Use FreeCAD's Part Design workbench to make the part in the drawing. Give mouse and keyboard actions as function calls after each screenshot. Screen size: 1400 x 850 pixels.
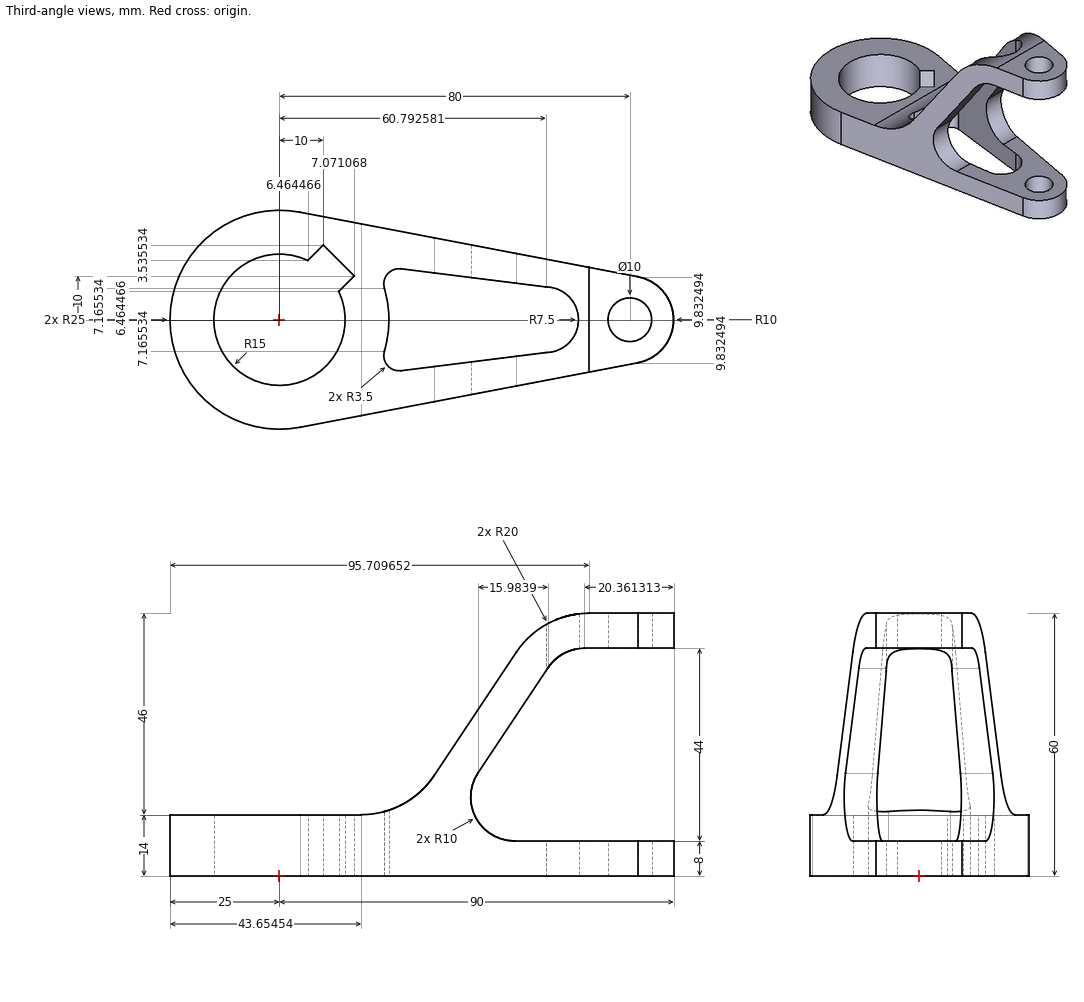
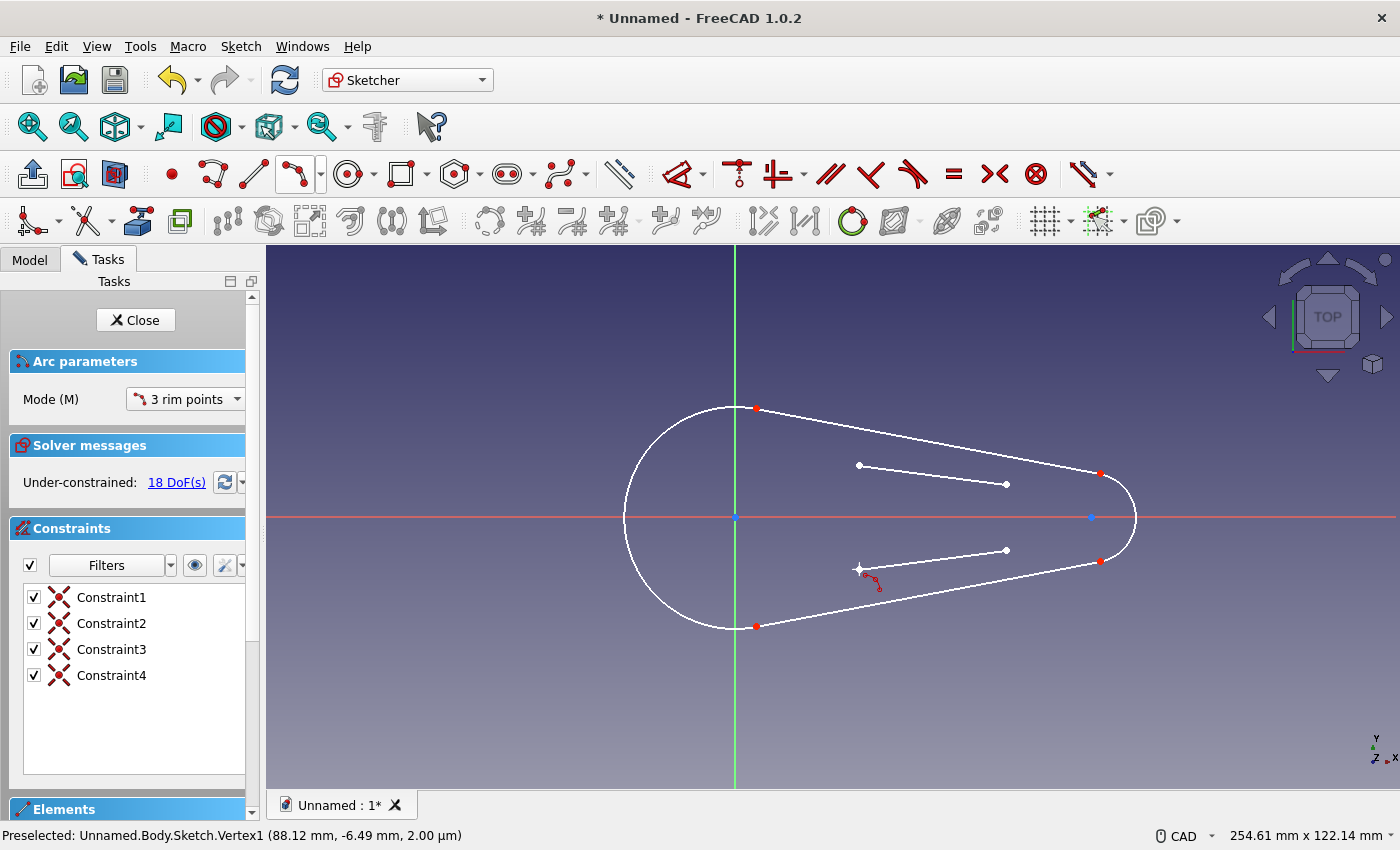
click(1006, 485)
click(1006, 551)
click(1033, 537)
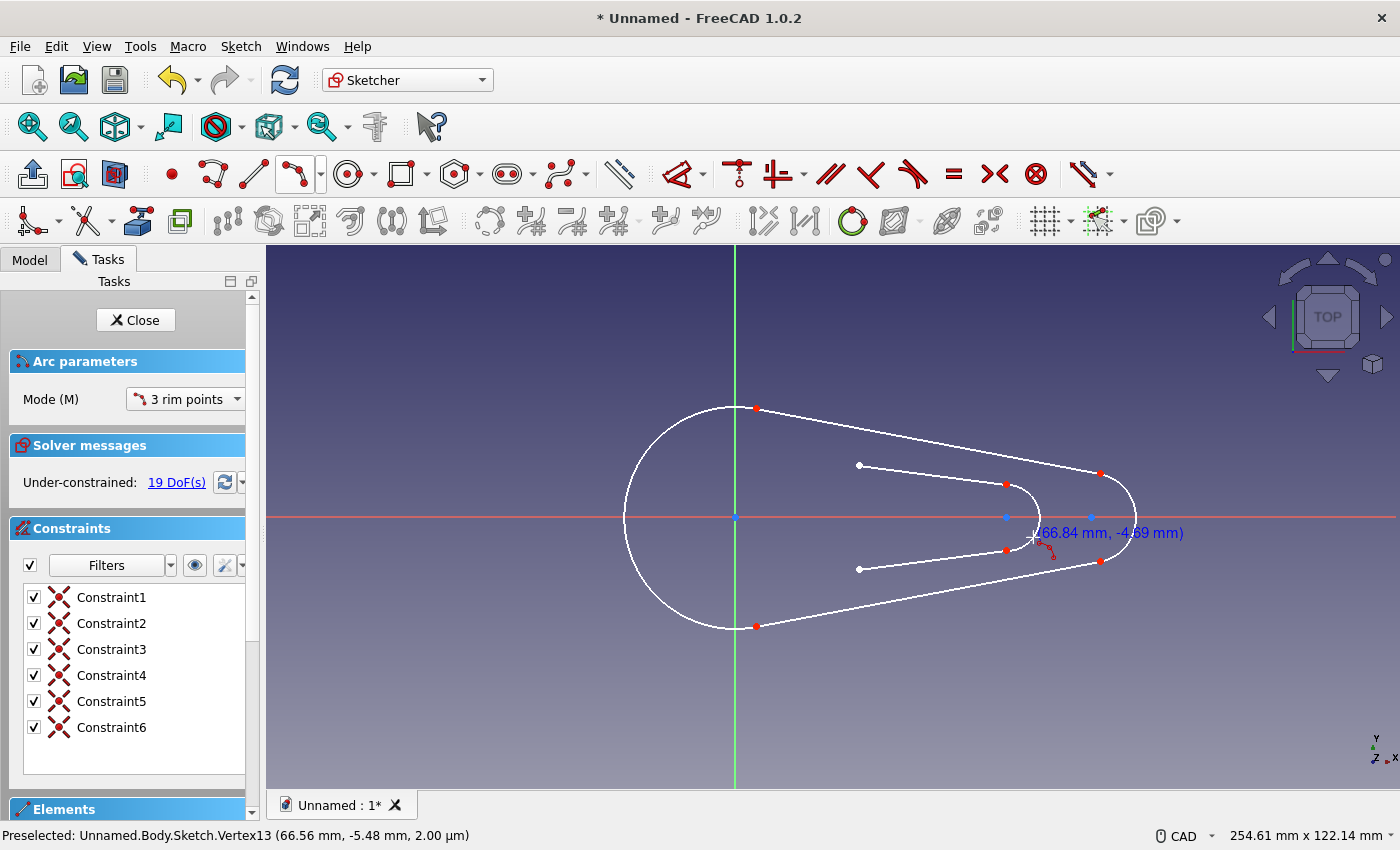
click(859, 570)
click(842, 549)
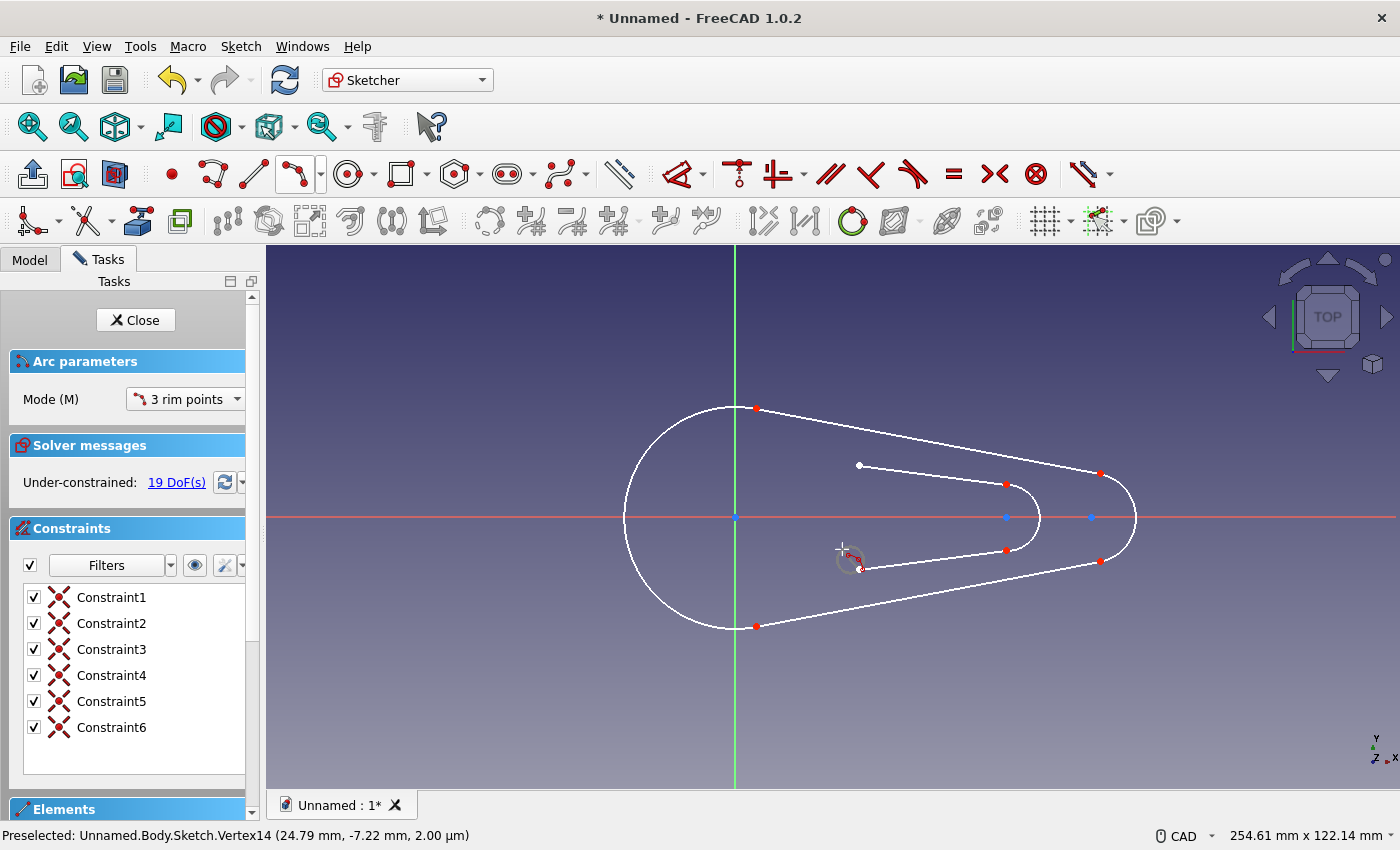
scroll(845, 564, up, 5)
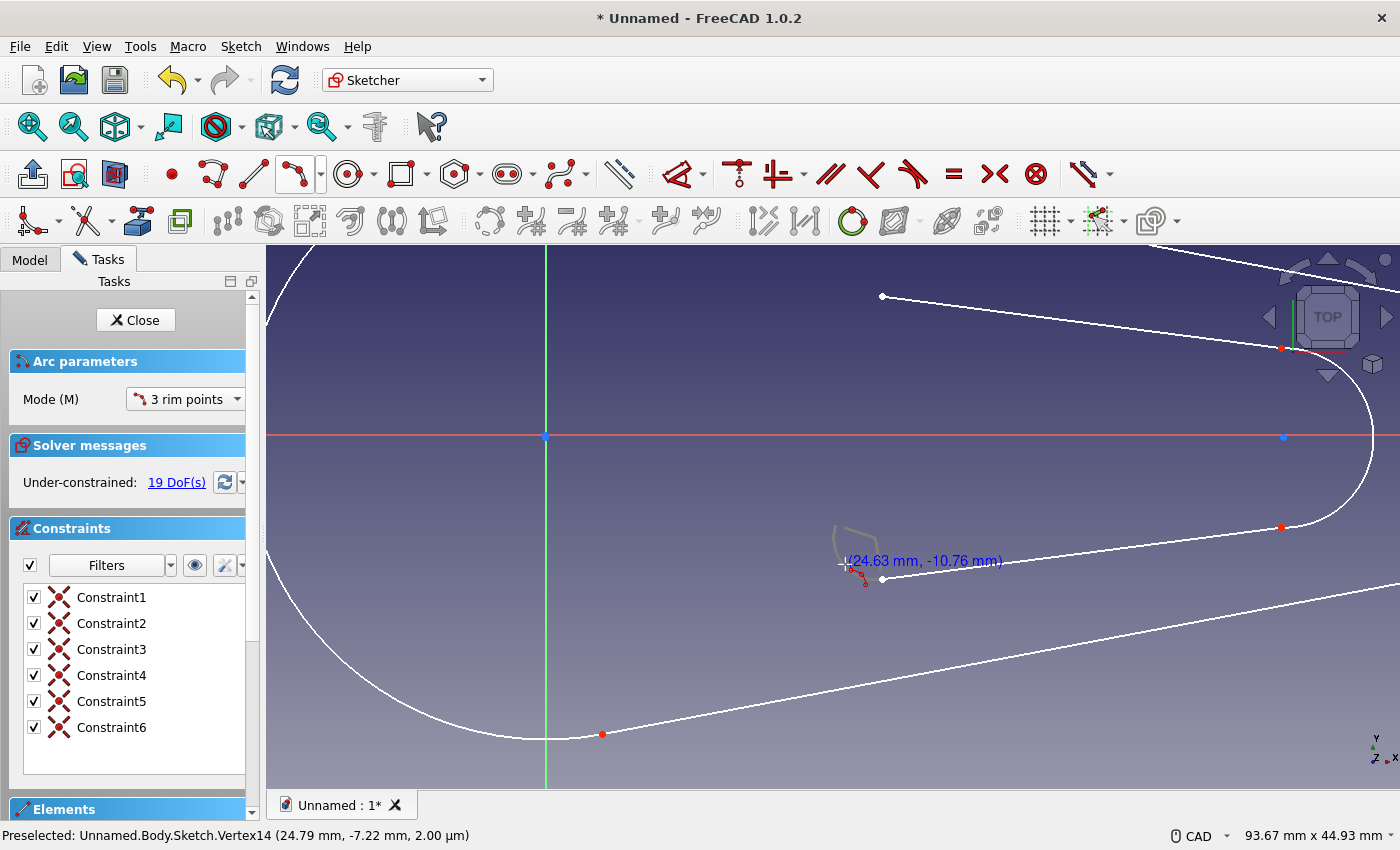
click(844, 562)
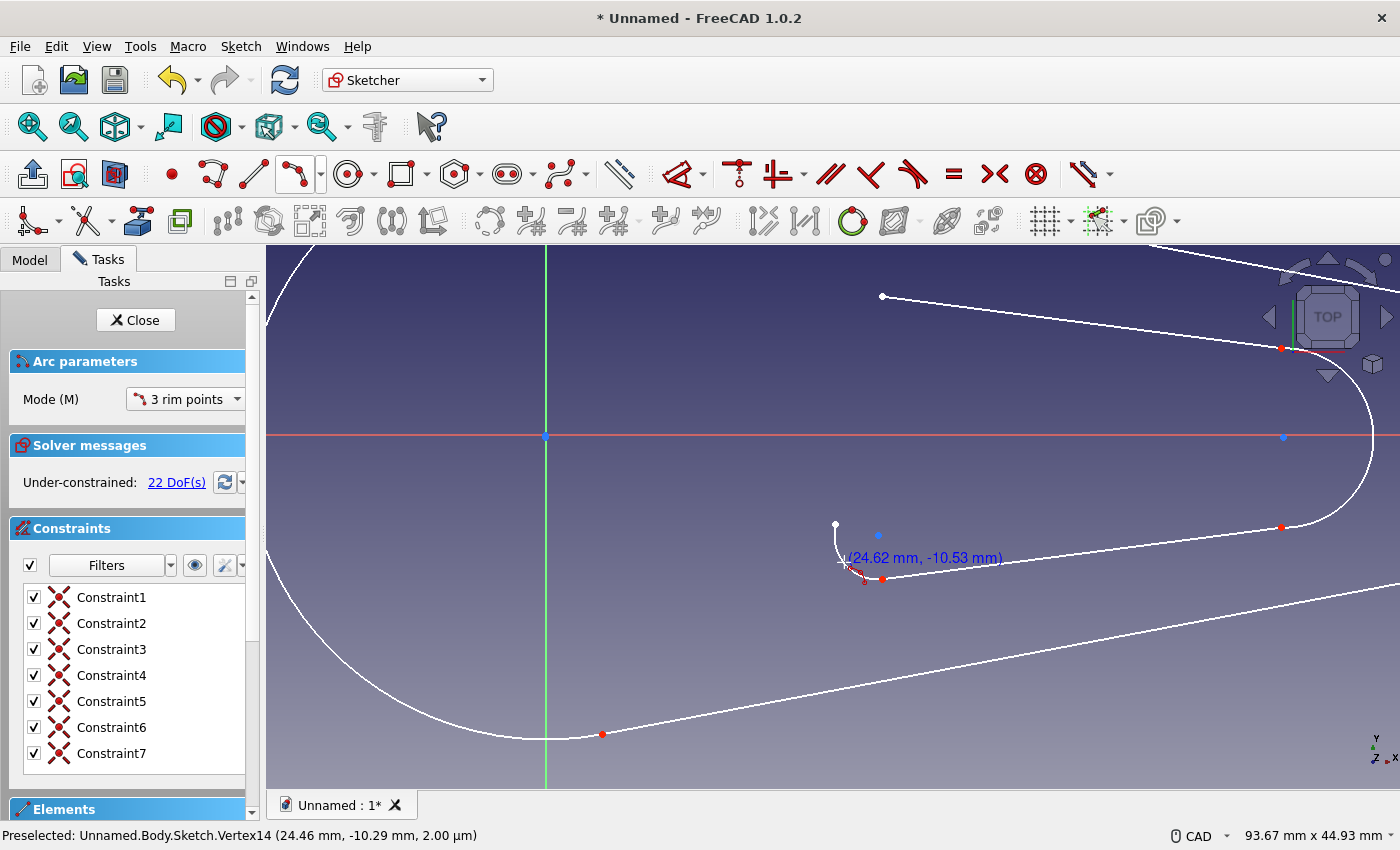
click(836, 525)
click(836, 349)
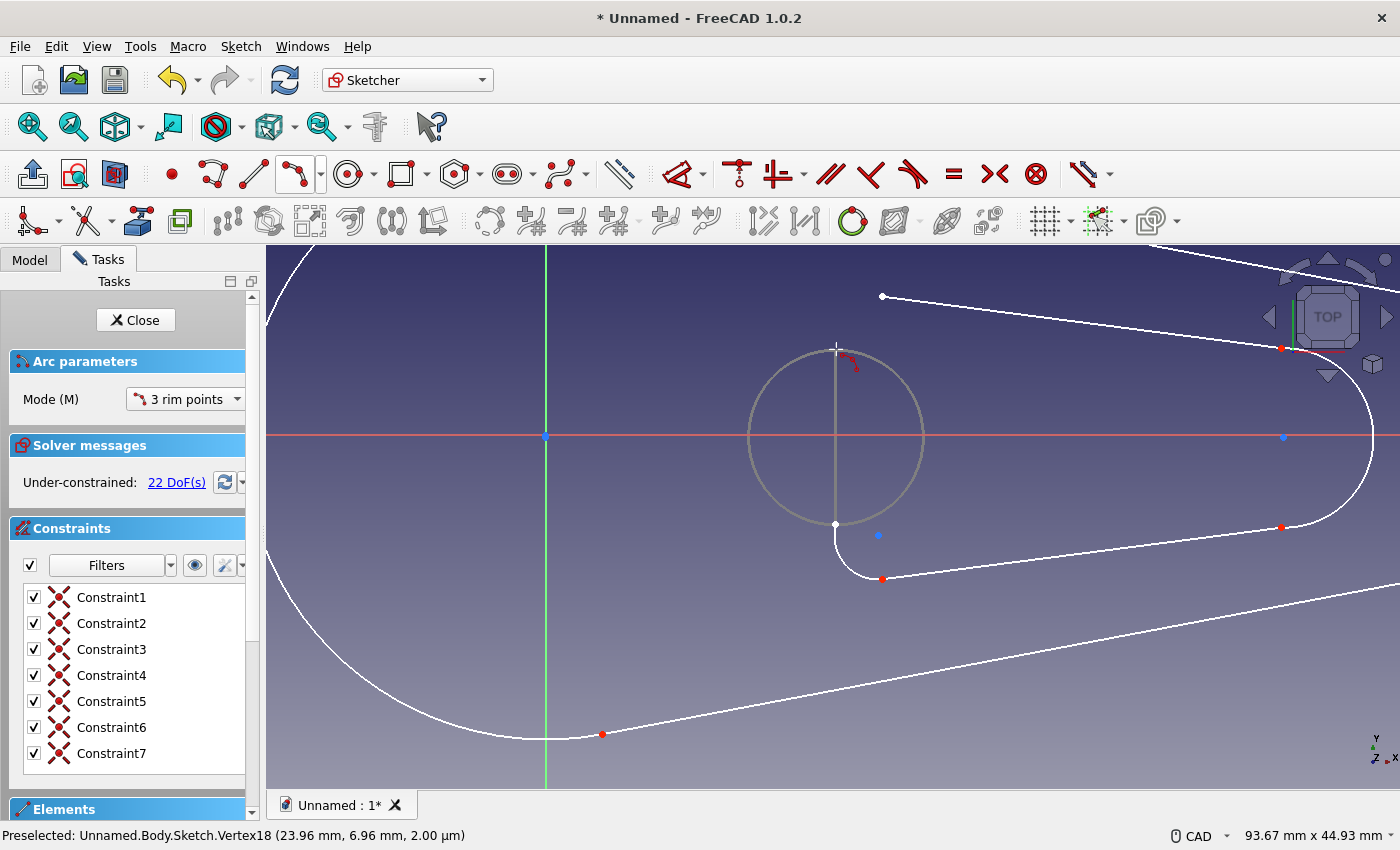
scroll(848, 453, up, 2)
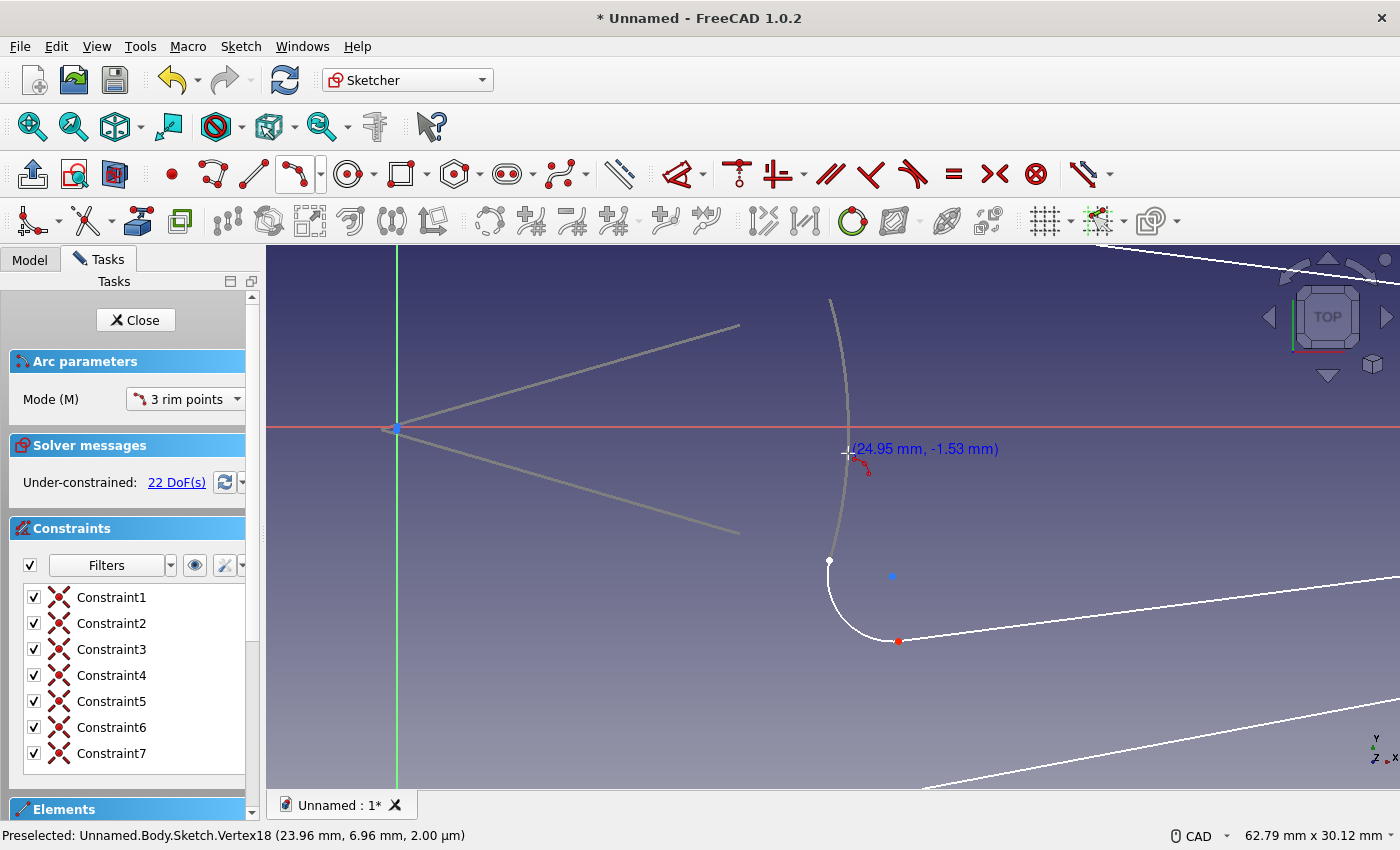
click(848, 453)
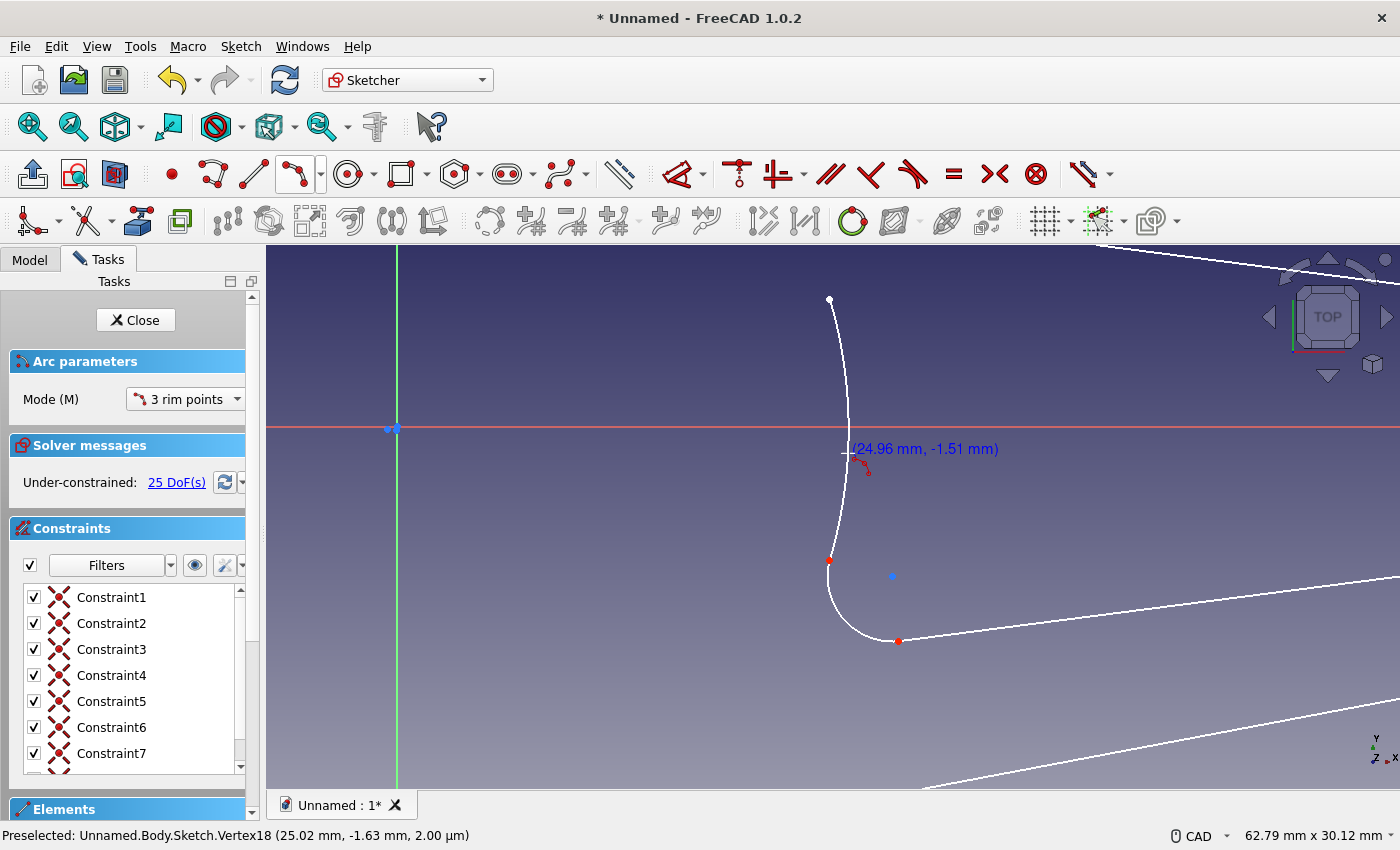
scroll(670, 556, down, 6)